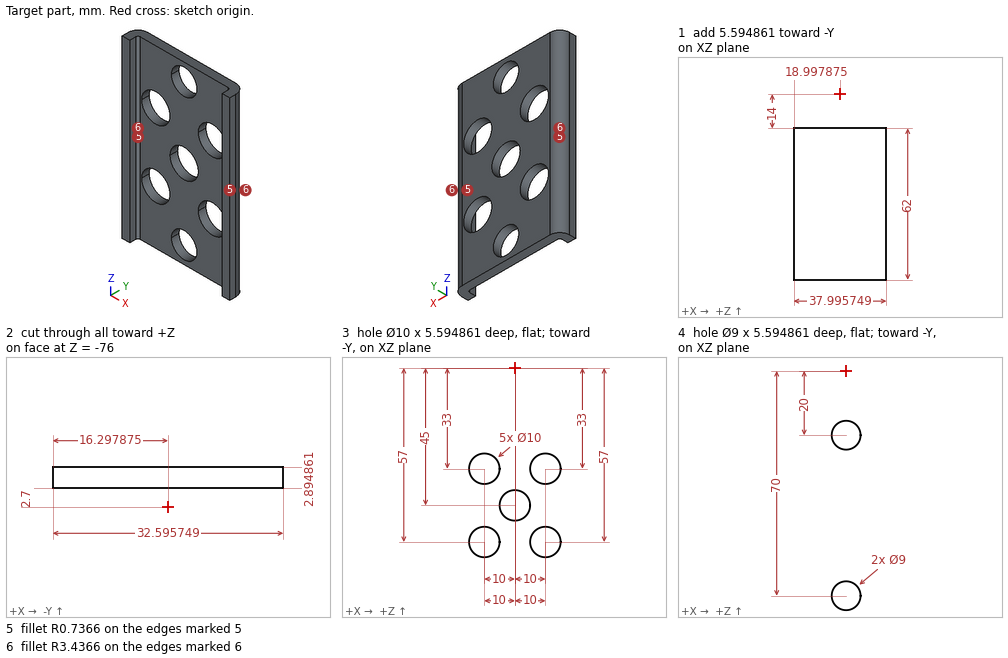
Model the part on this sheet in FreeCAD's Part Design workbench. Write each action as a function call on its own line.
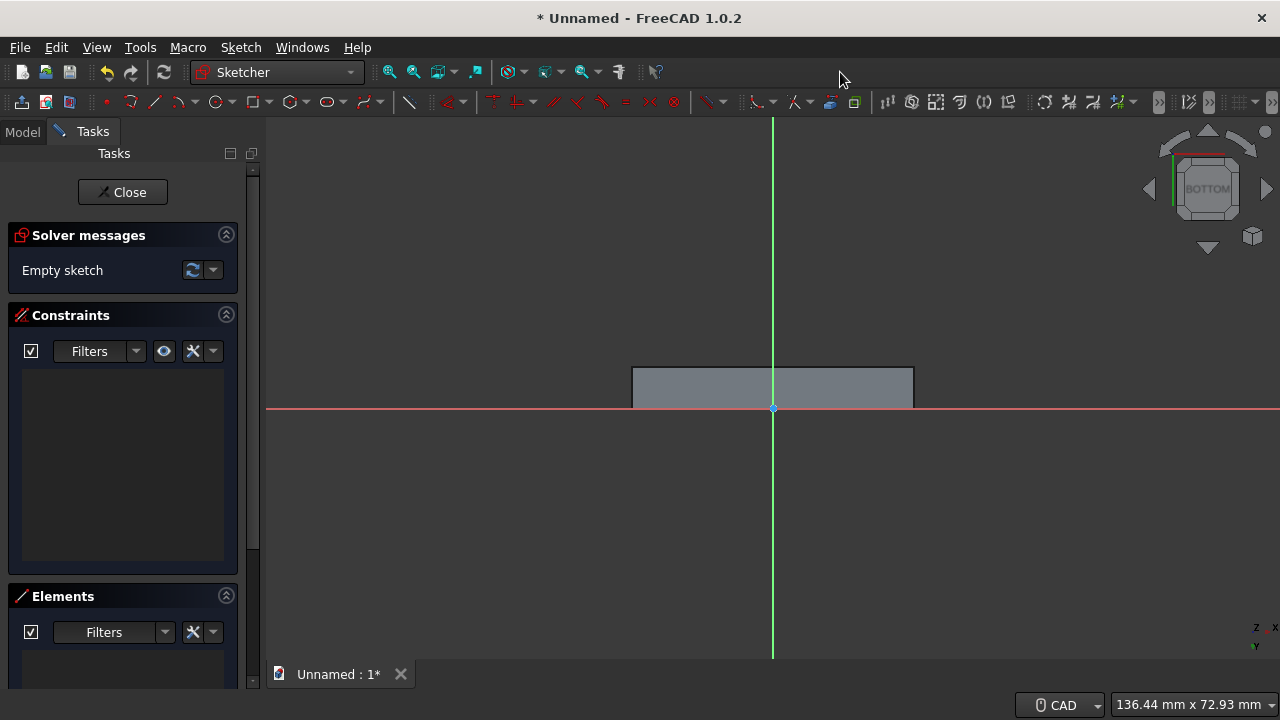
scroll(829, 388, up, 4)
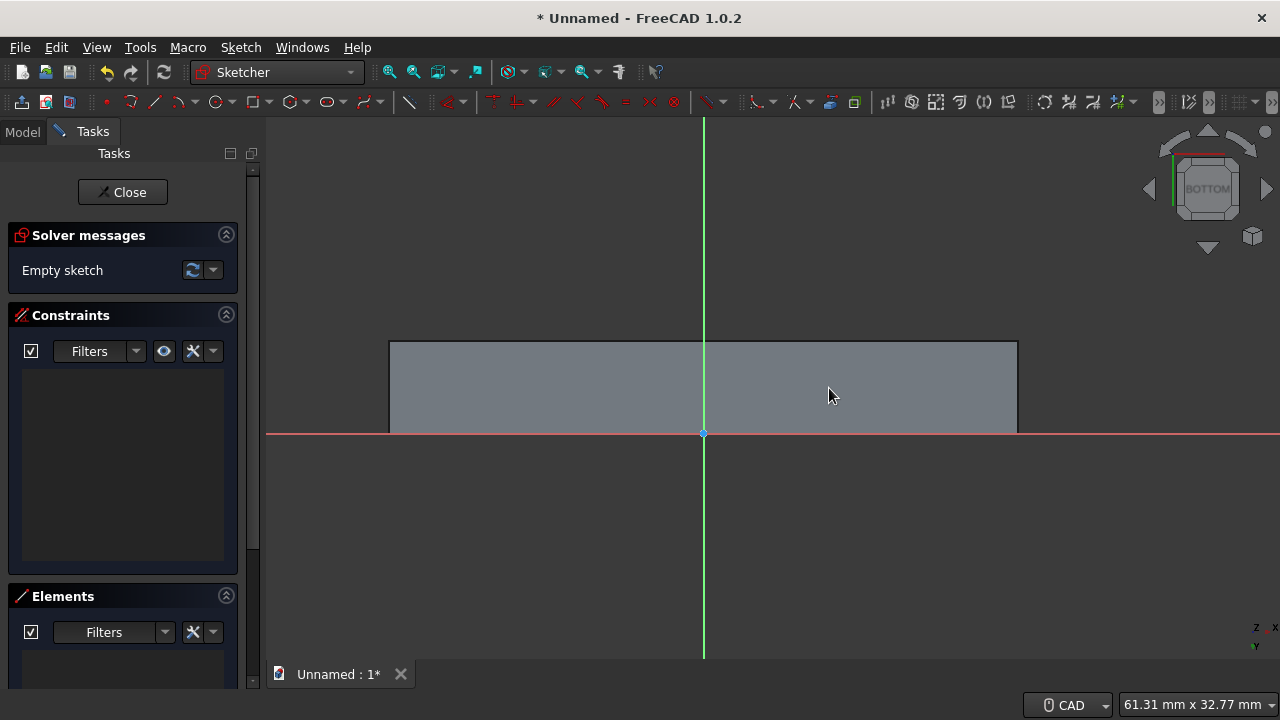
key(g)
key(r)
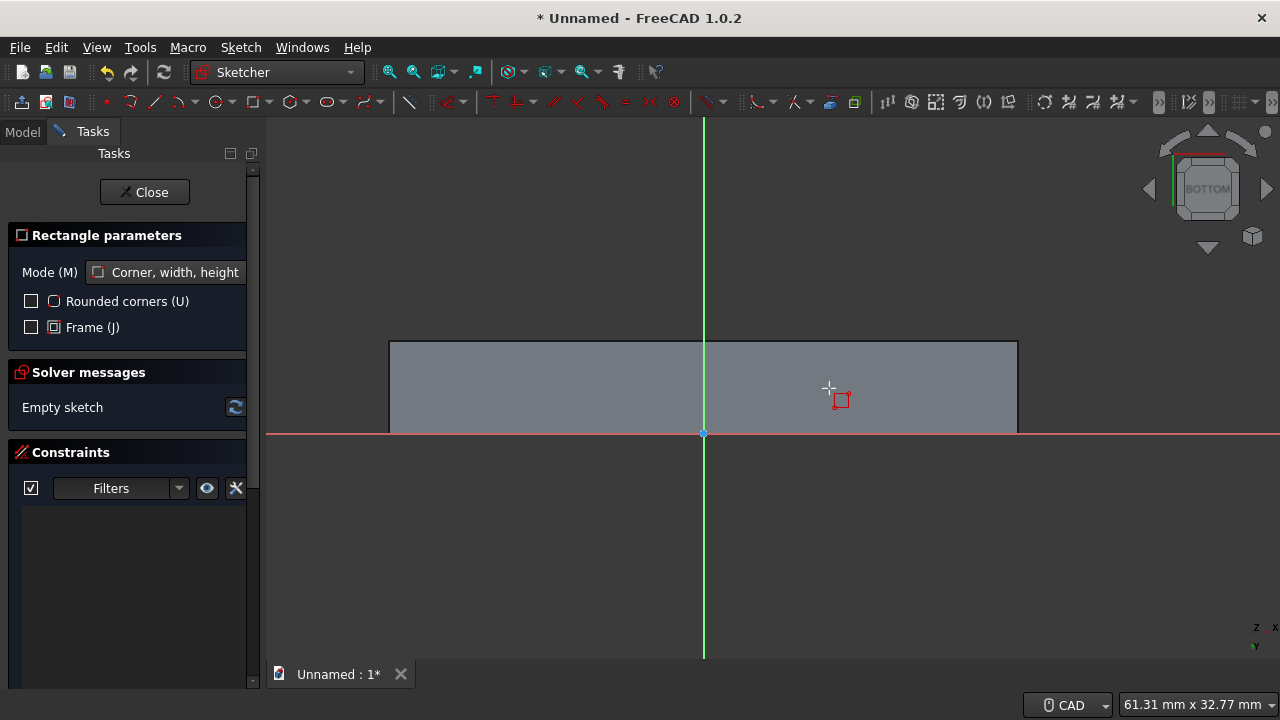
click(434, 341)
move(973, 389)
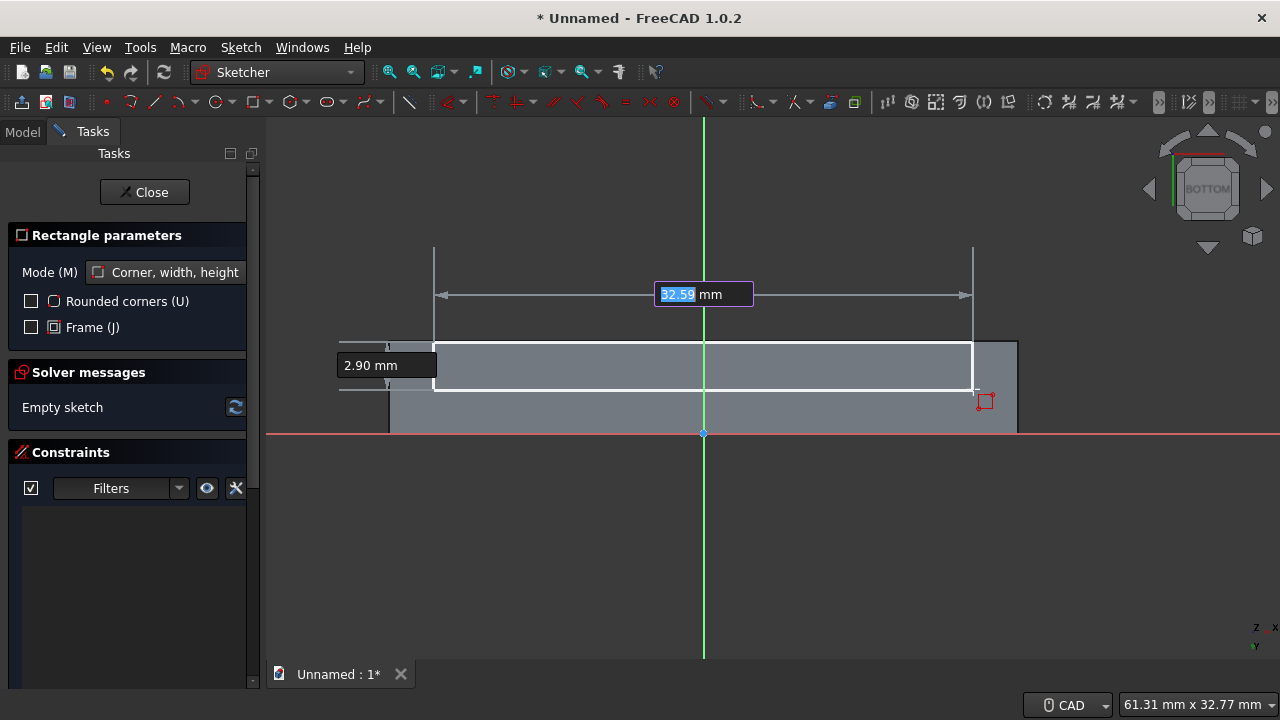
text(32.595749)
key(Tab)
text(2.894861)
key(Return)
key(Escape)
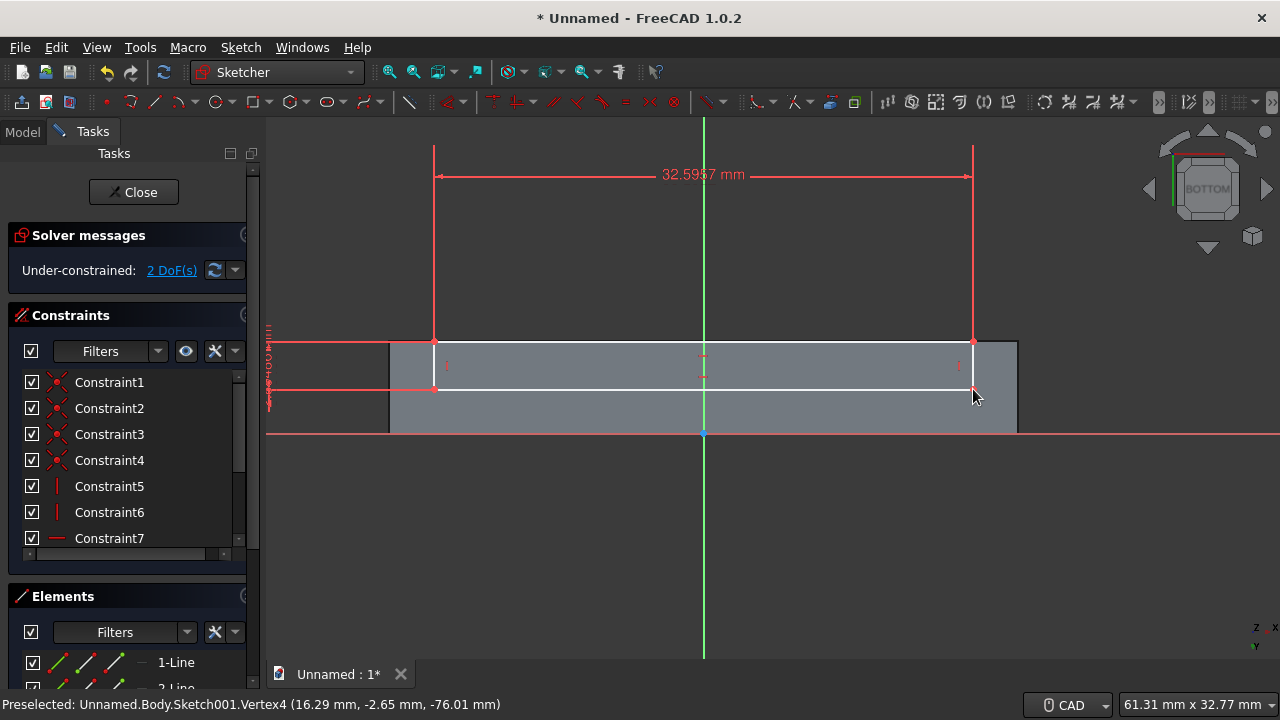
key(d)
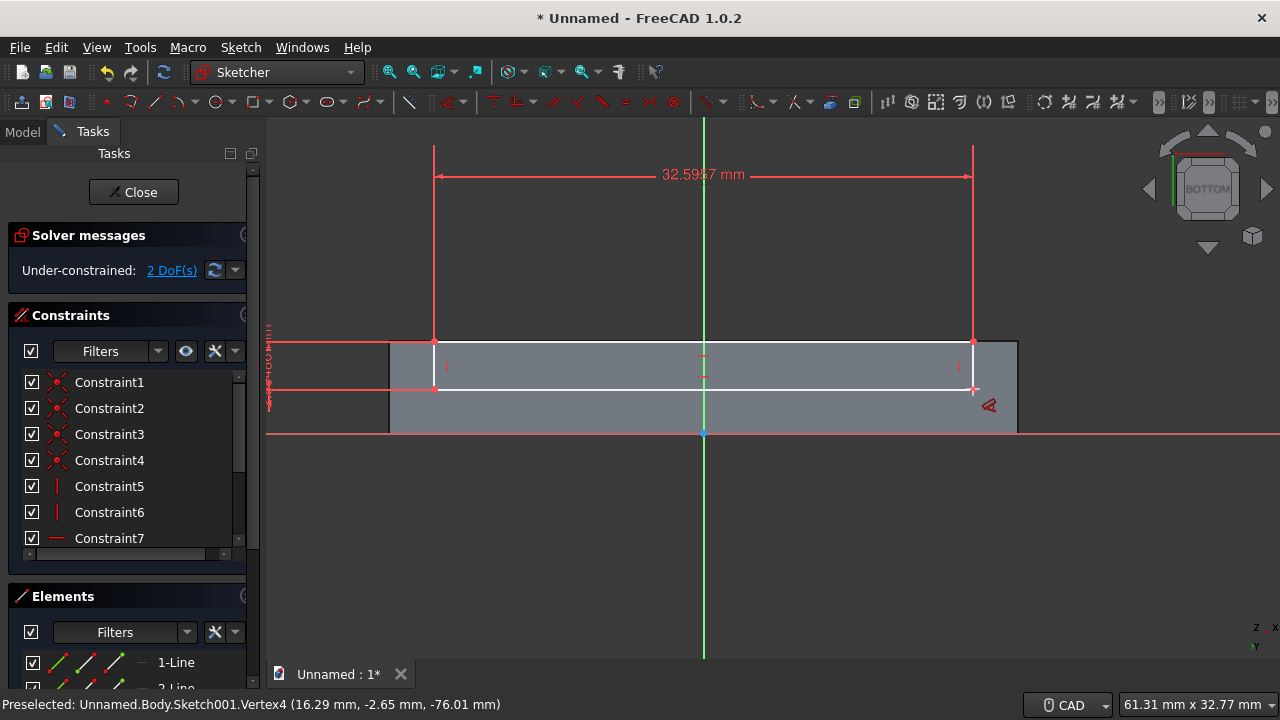
click(434, 390)
click(400, 412)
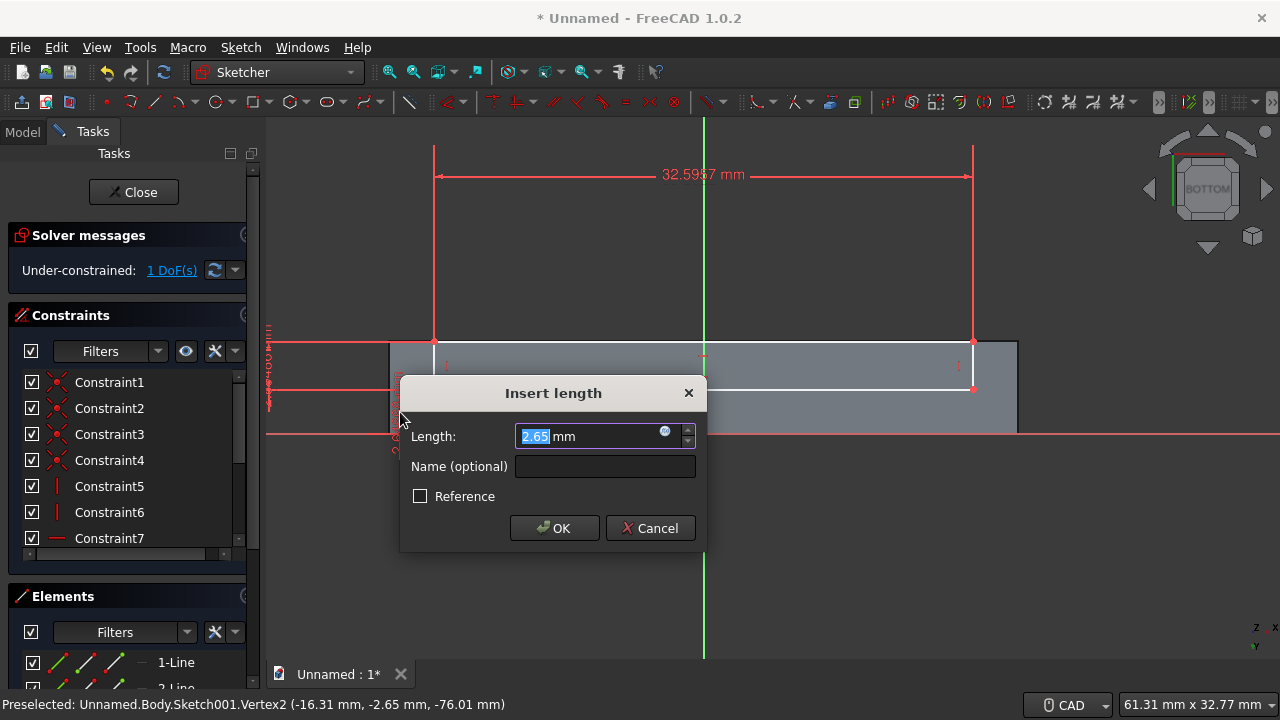
text(2.7)
key(Return)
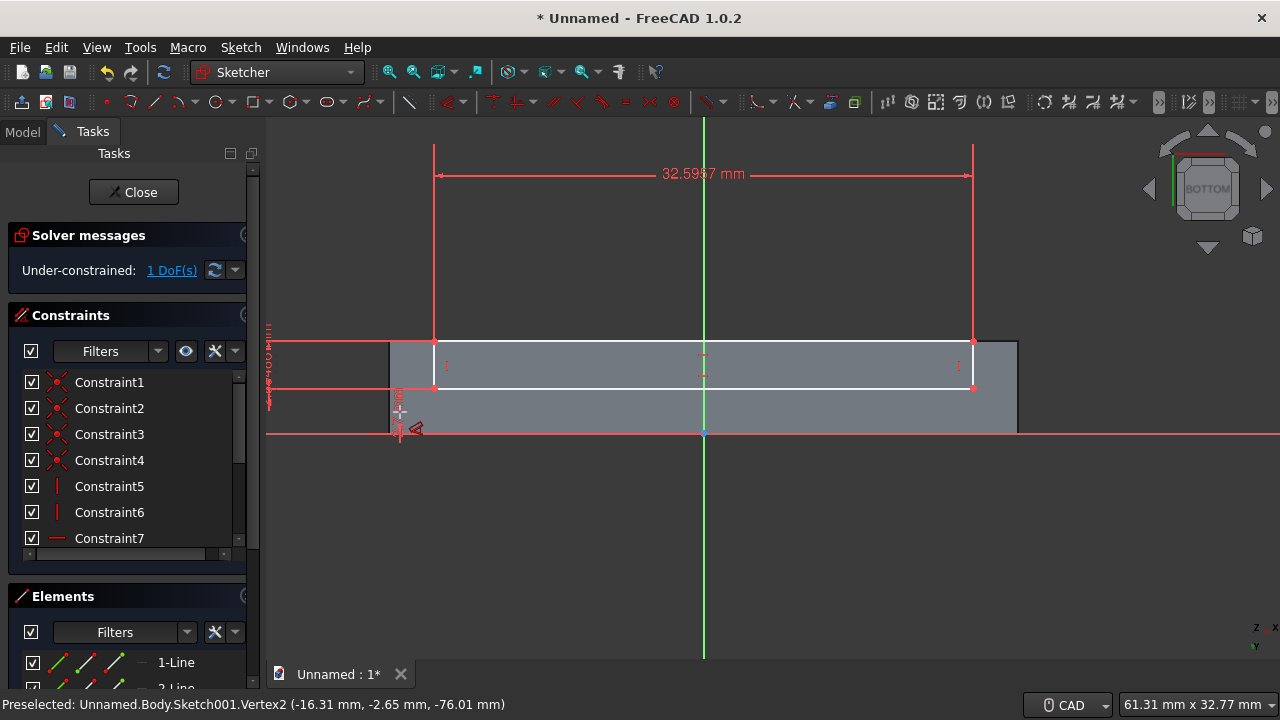
click(434, 341)
click(569, 307)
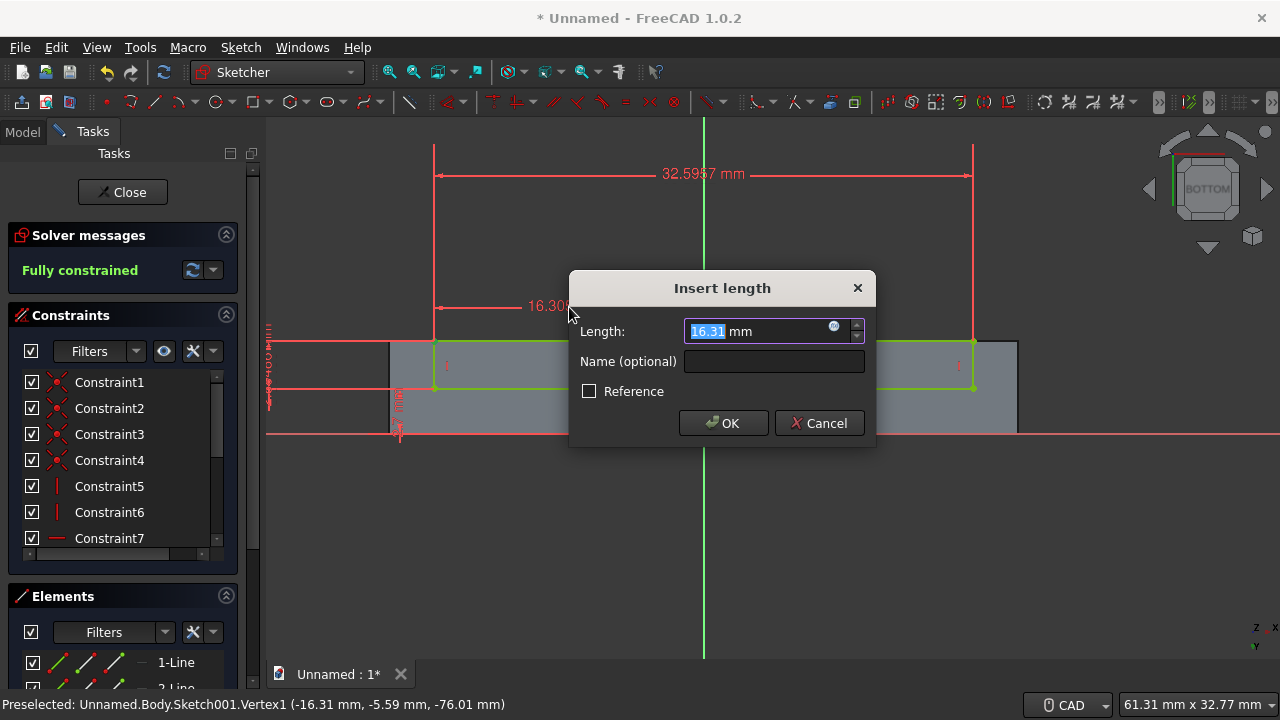
text(16.297875)
key(Return)
key(Escape)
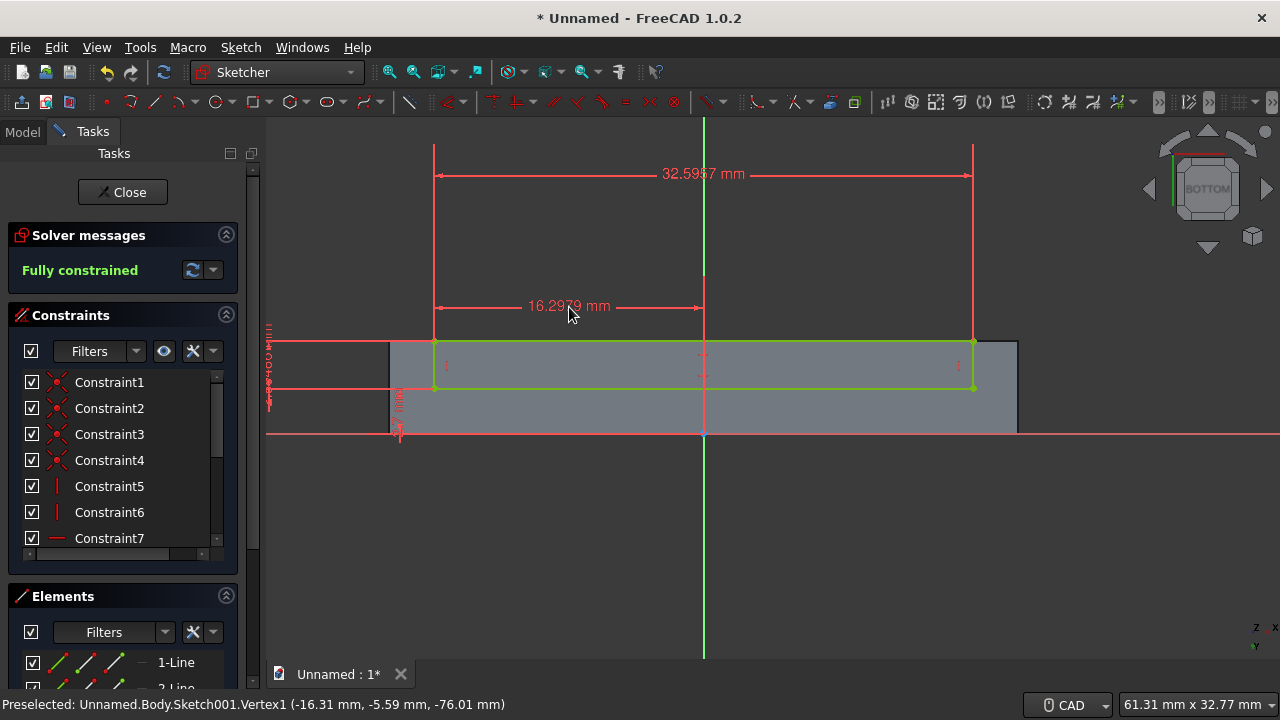
click(123, 192)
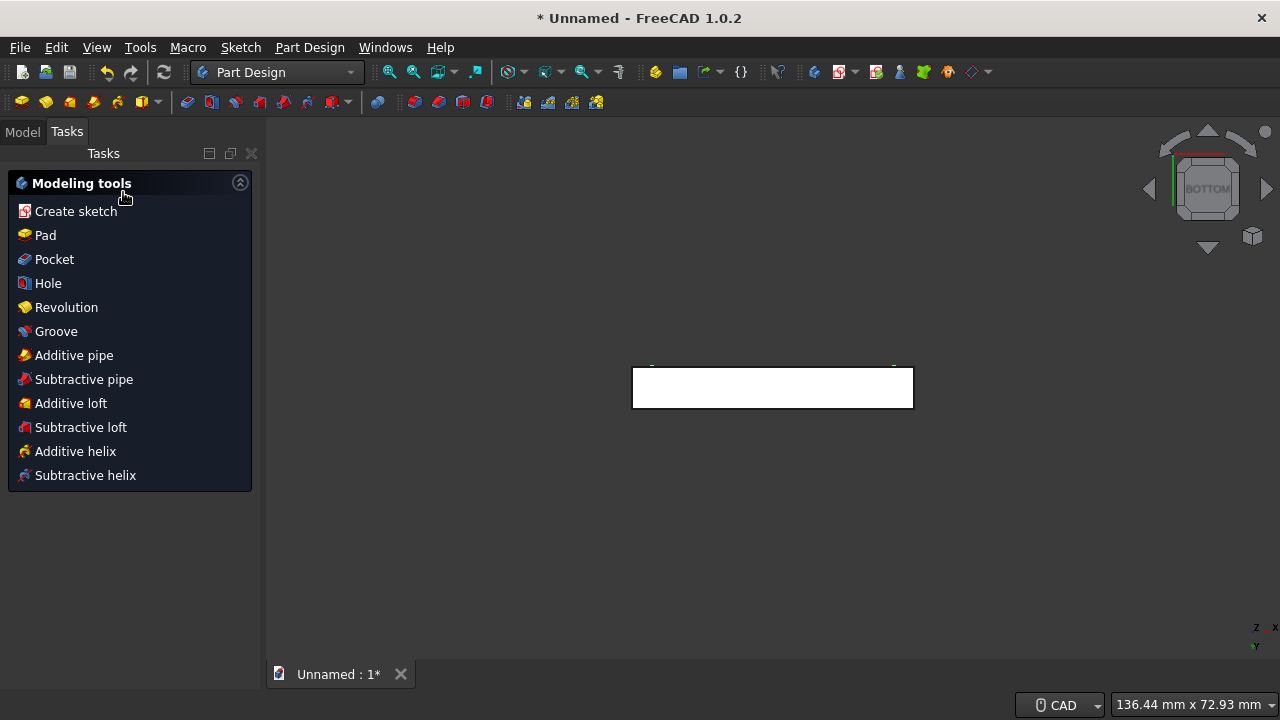
click(188, 102)